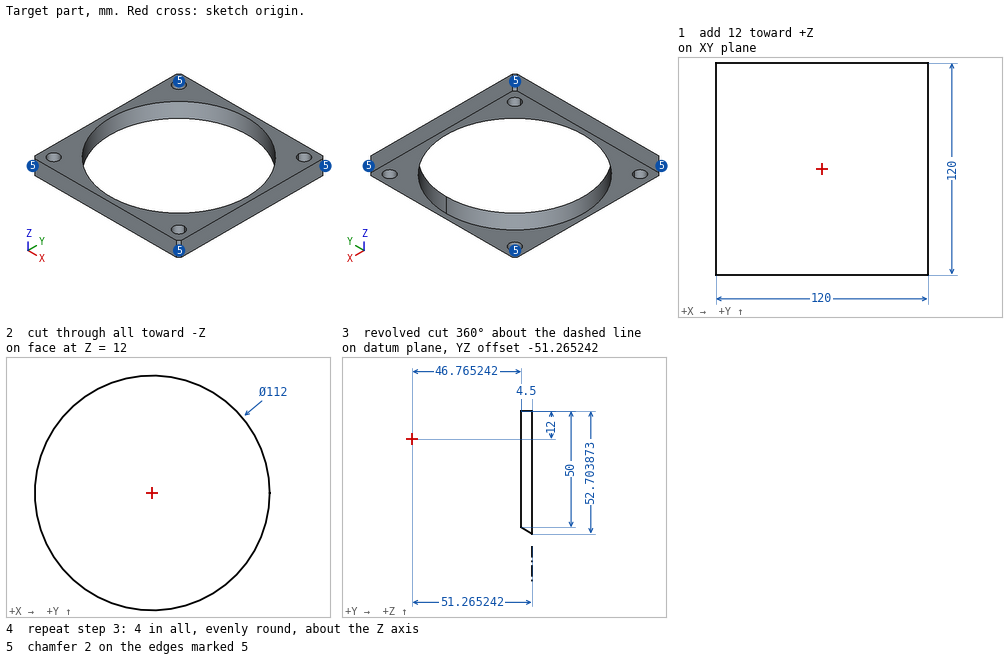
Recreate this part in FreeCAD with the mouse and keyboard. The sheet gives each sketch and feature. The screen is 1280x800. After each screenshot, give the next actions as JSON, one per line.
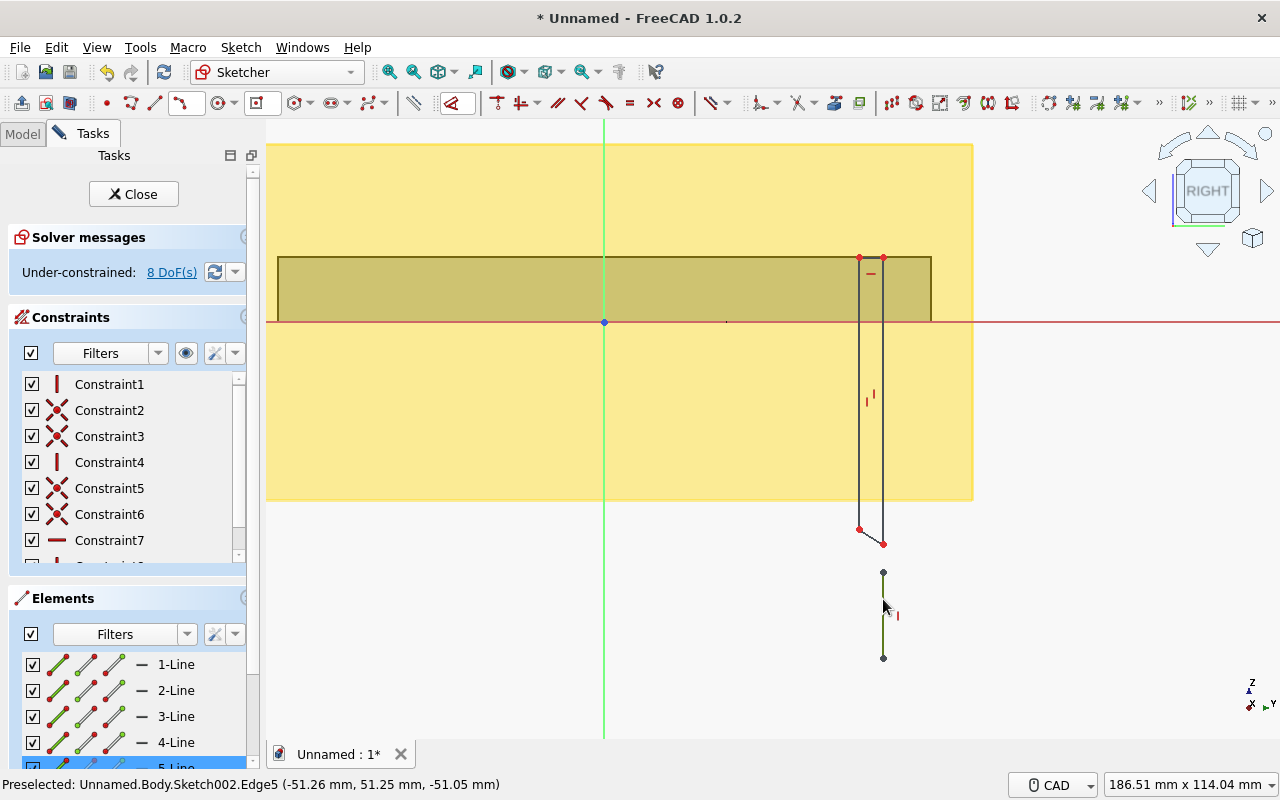
{"action": "key", "text": "g n"}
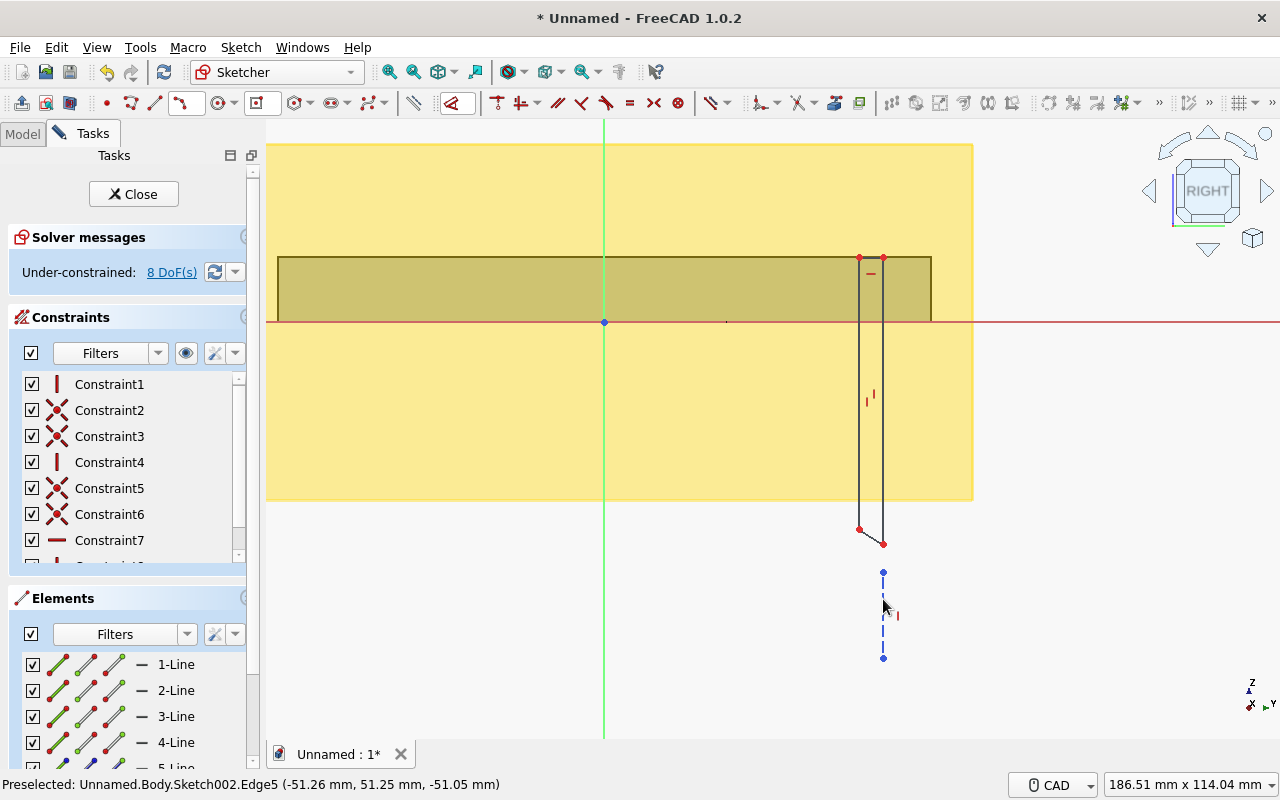
{"action": "key", "text": "d"}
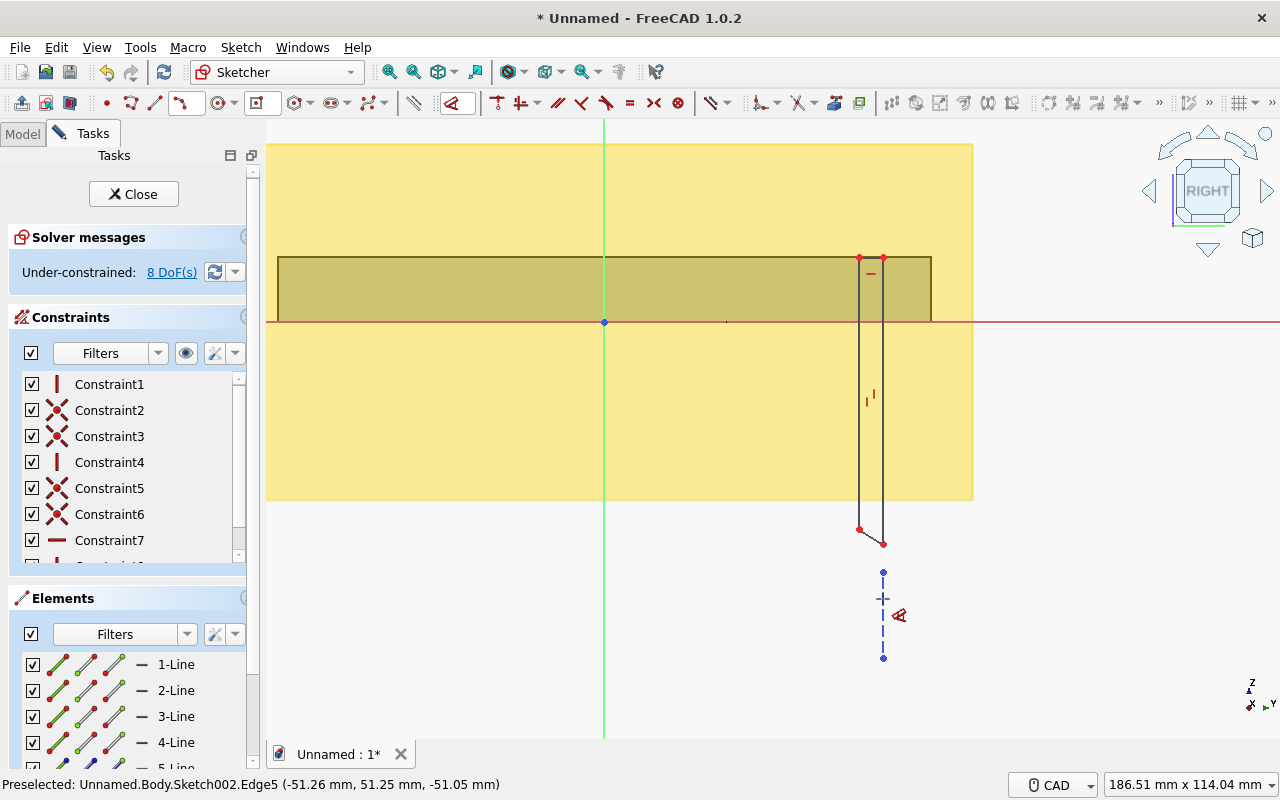
{"action": "left_click", "coordinate": [859, 340]}
{"action": "left_click", "coordinate": [825, 394]}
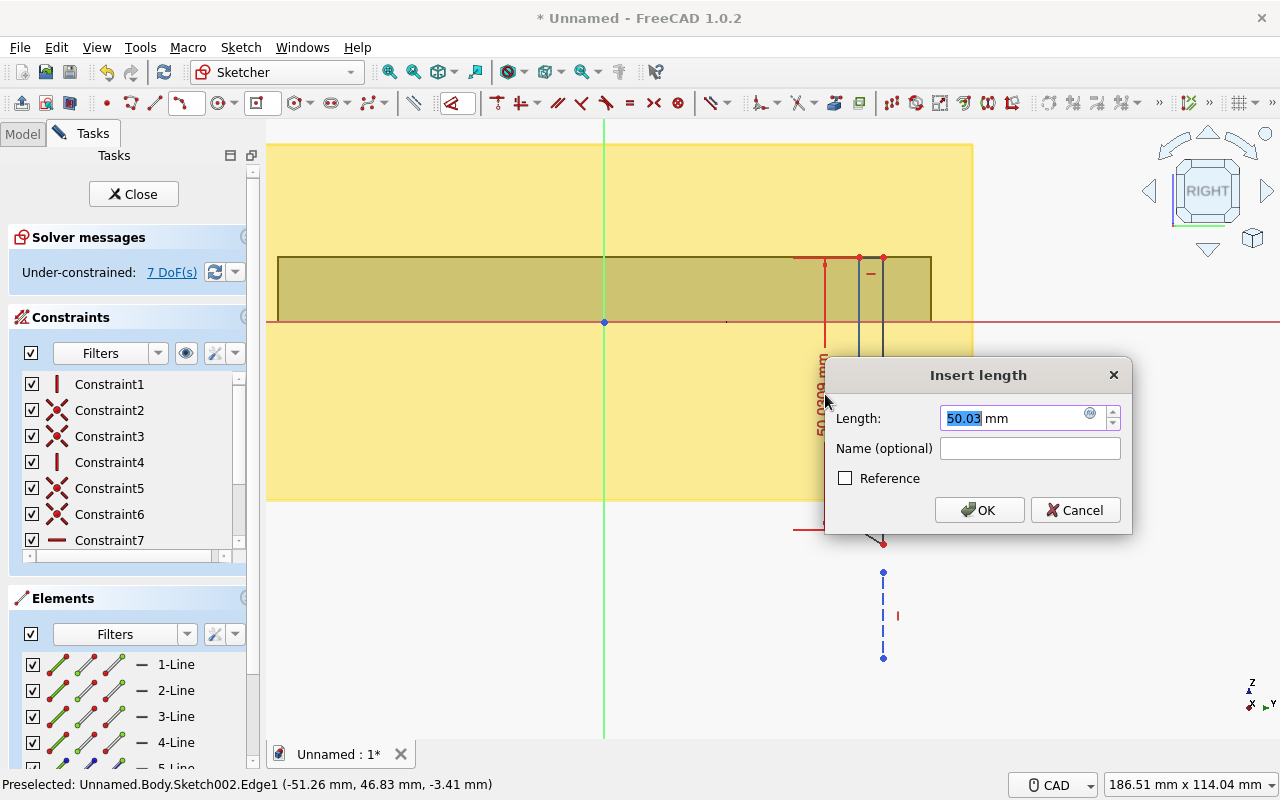
{"action": "type", "text": "50"}
{"action": "key", "text": "Return"}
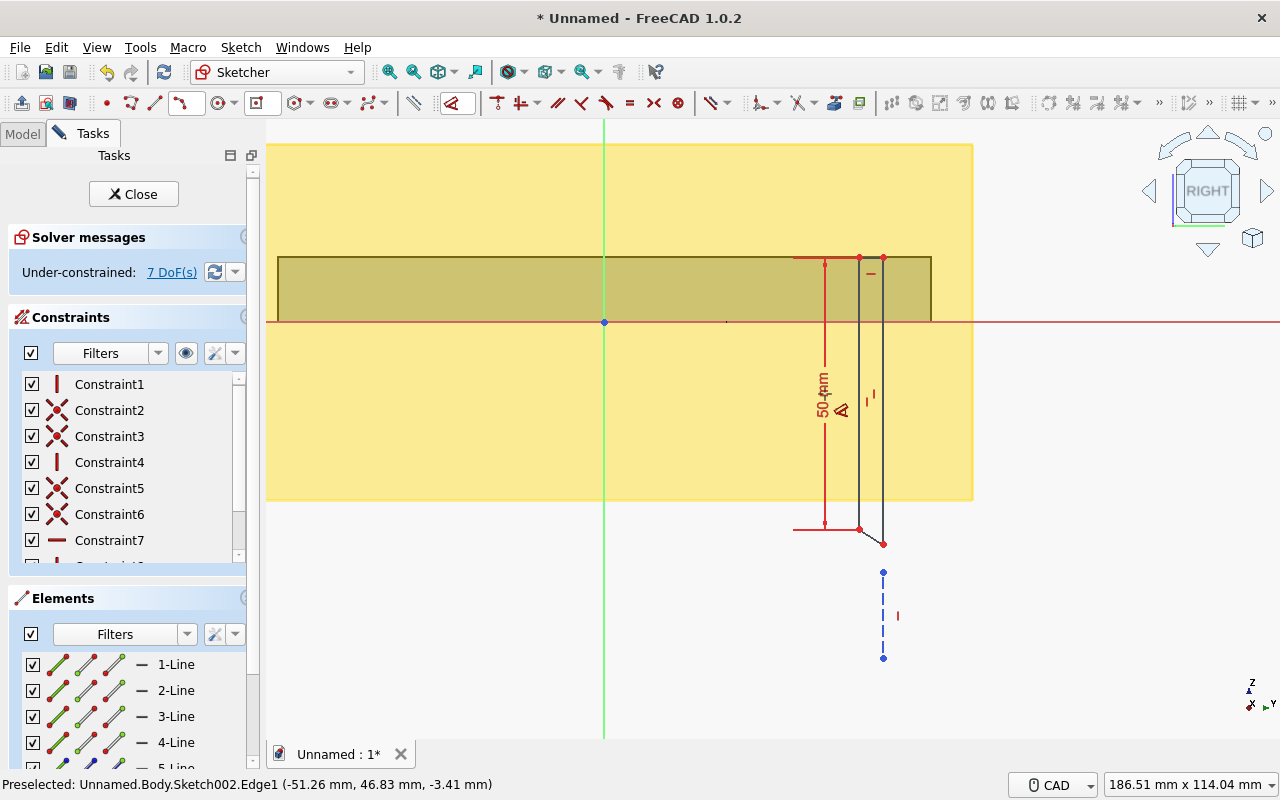
{"action": "scroll", "coordinate": [873, 258], "scroll_direction": "up", "scroll_amount": 3}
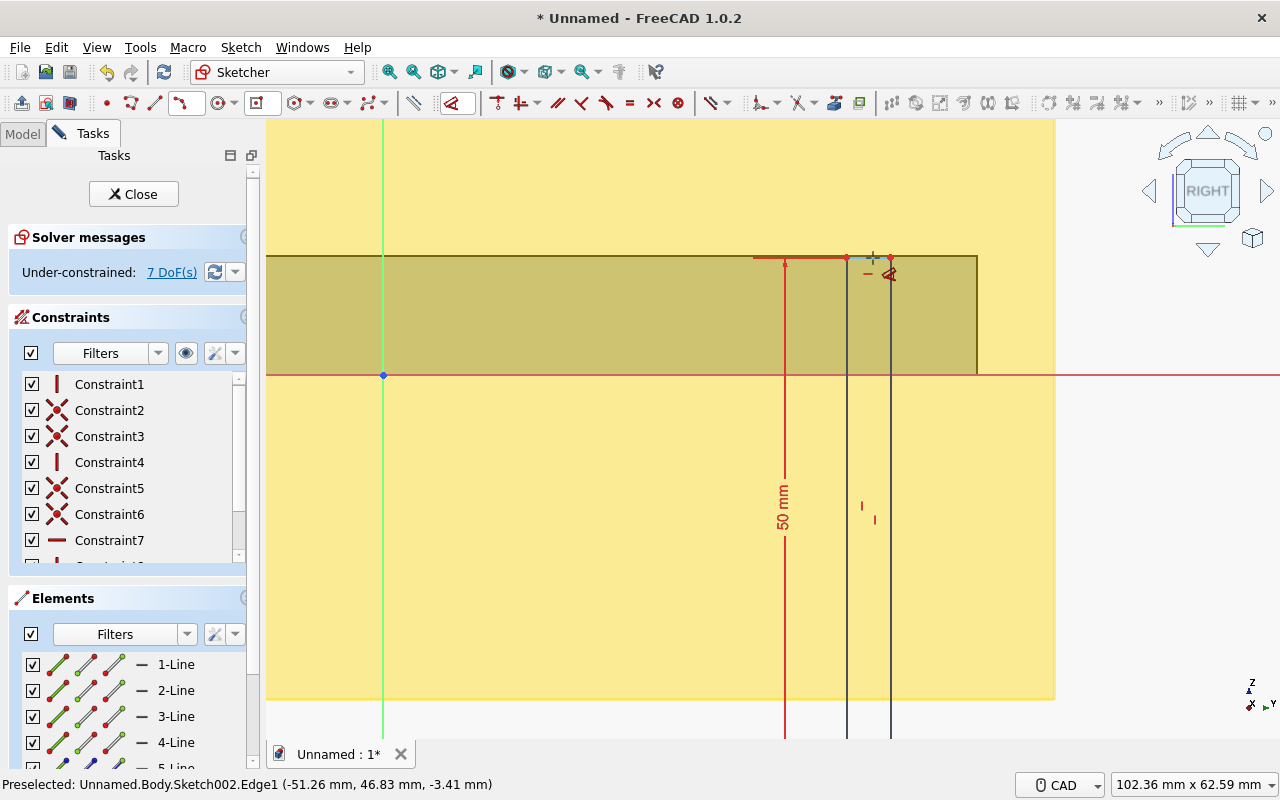
{"action": "left_click", "coordinate": [873, 258]}
{"action": "left_click", "coordinate": [869, 224]}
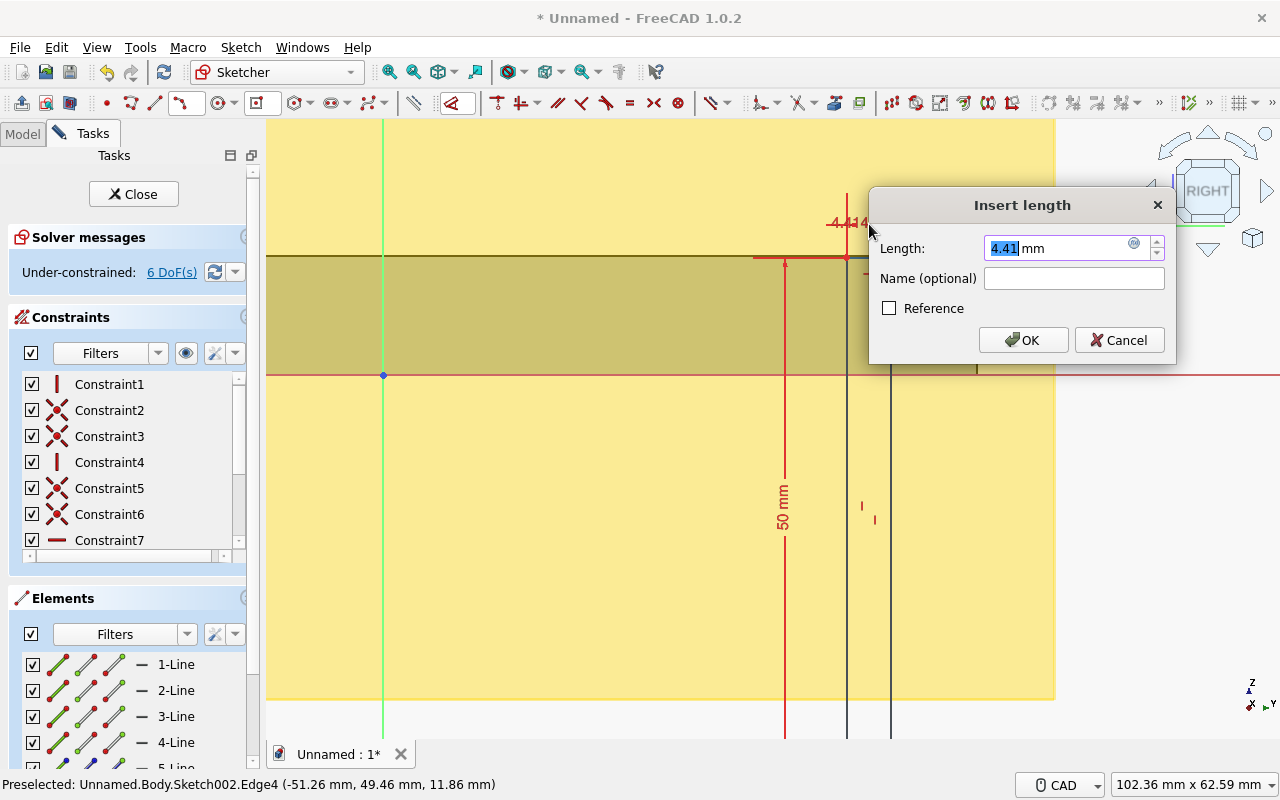
{"action": "type", "text": "4.5"}
{"action": "key", "text": "Return"}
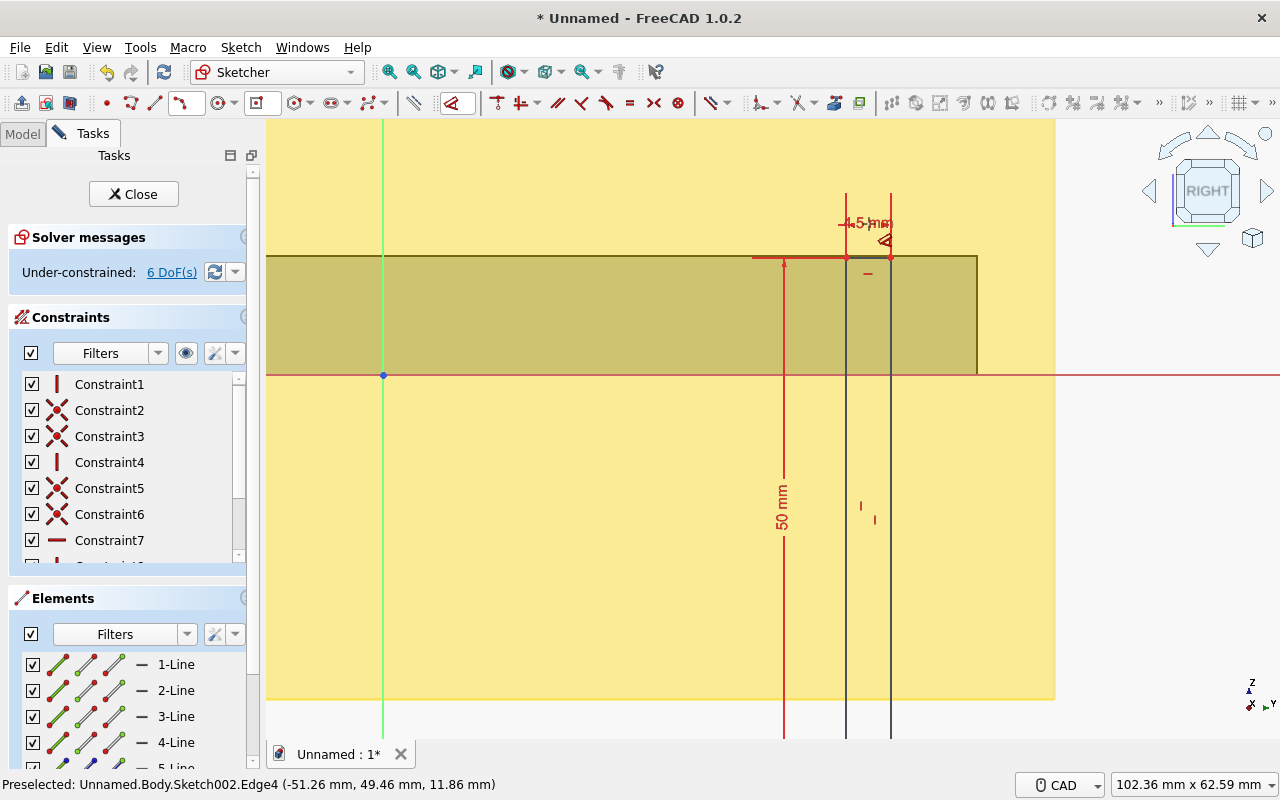
{"action": "left_click", "coordinate": [846, 258]}
{"action": "left_click", "coordinate": [349, 317]}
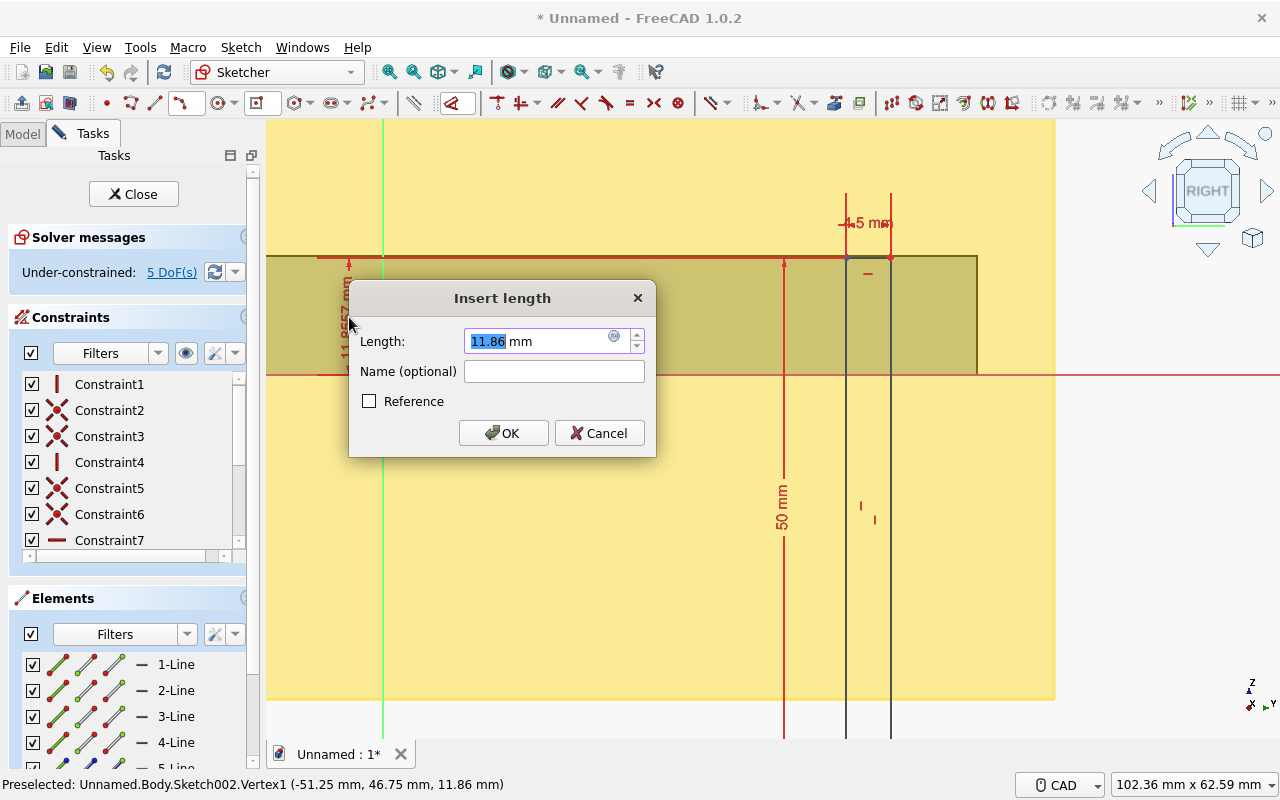
{"action": "type", "text": "12"}
{"action": "key", "text": "Return"}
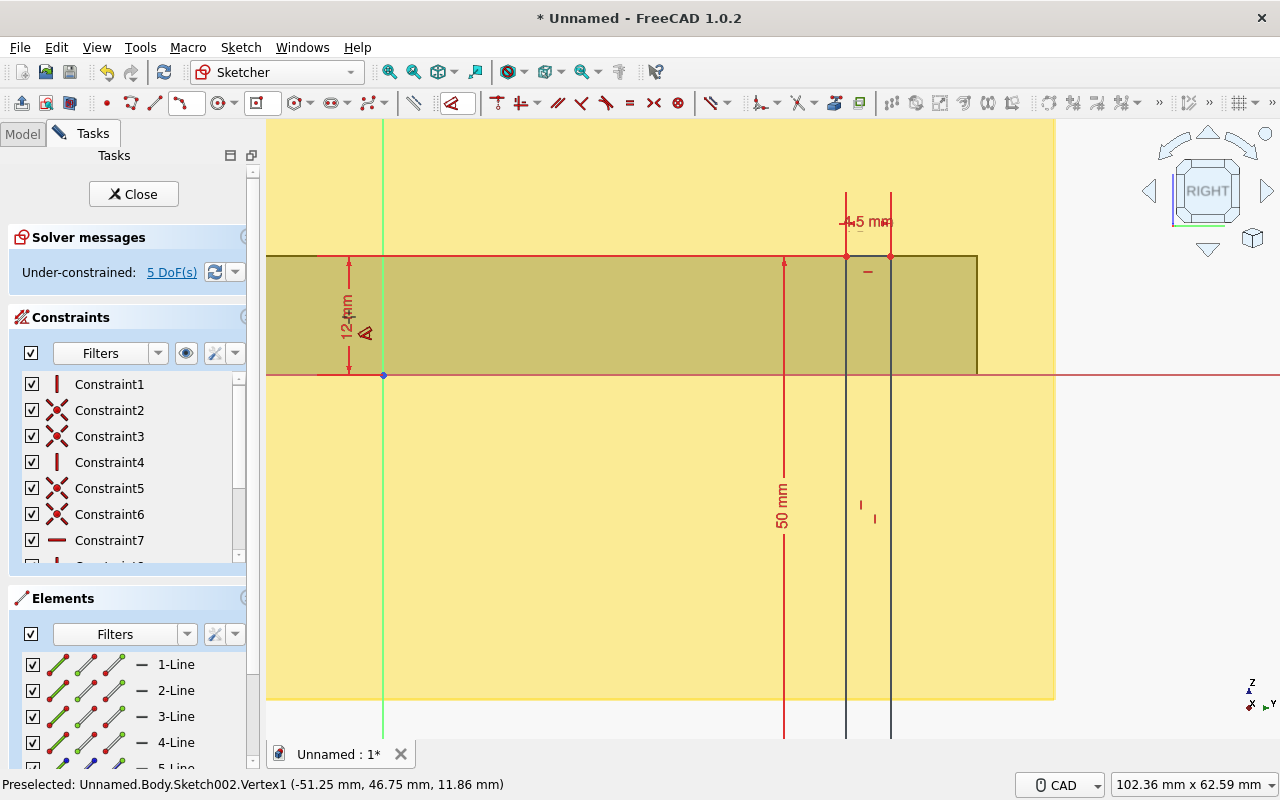
{"action": "left_click", "coordinate": [891, 623]}
{"action": "left_click", "coordinate": [925, 484]}